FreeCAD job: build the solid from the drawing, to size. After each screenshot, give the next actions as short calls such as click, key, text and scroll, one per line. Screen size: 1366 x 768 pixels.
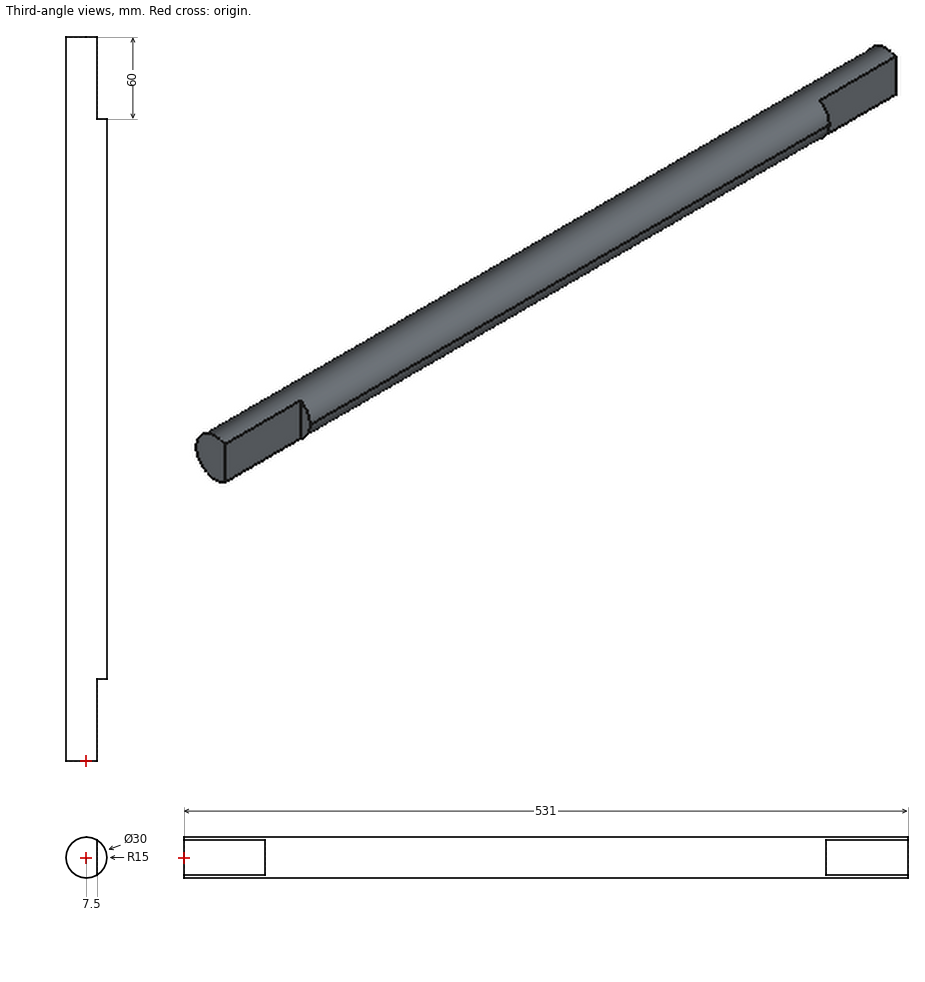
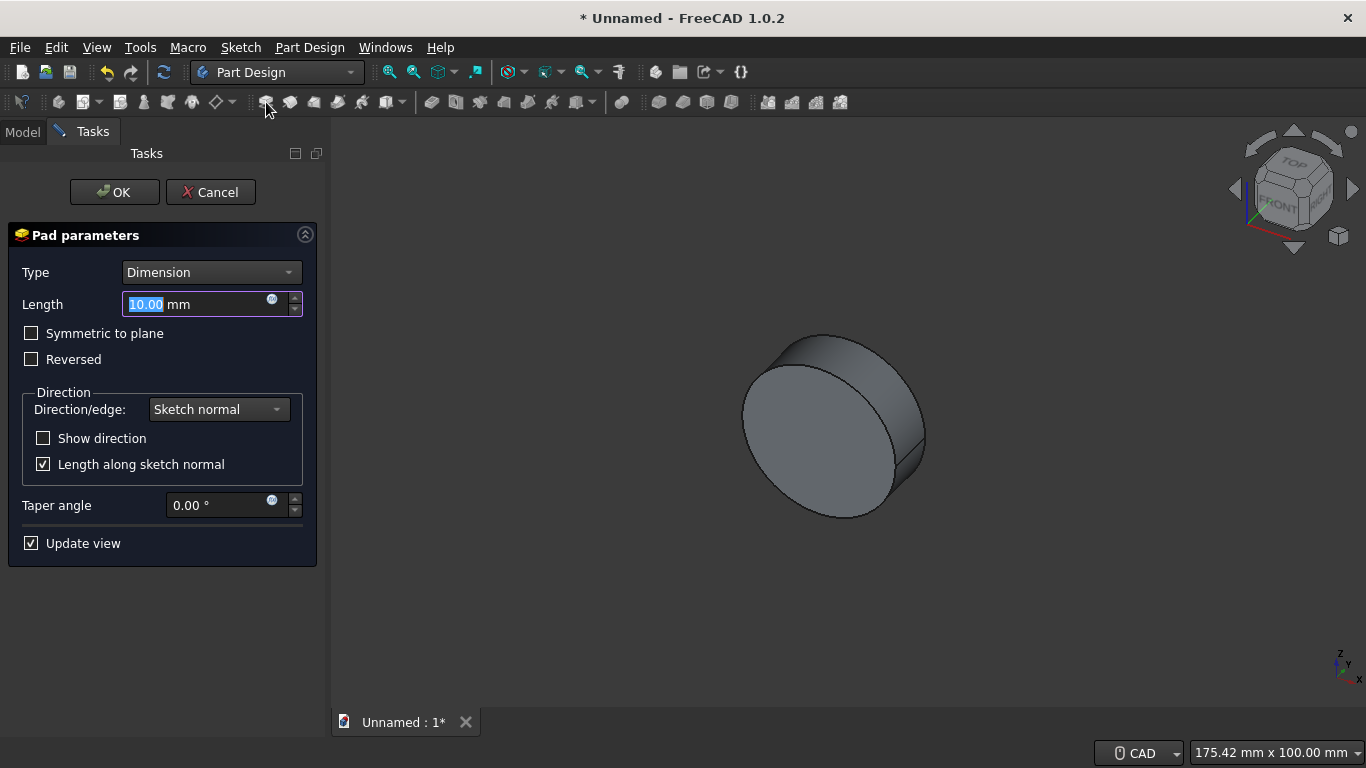
text(531)
key(Tab)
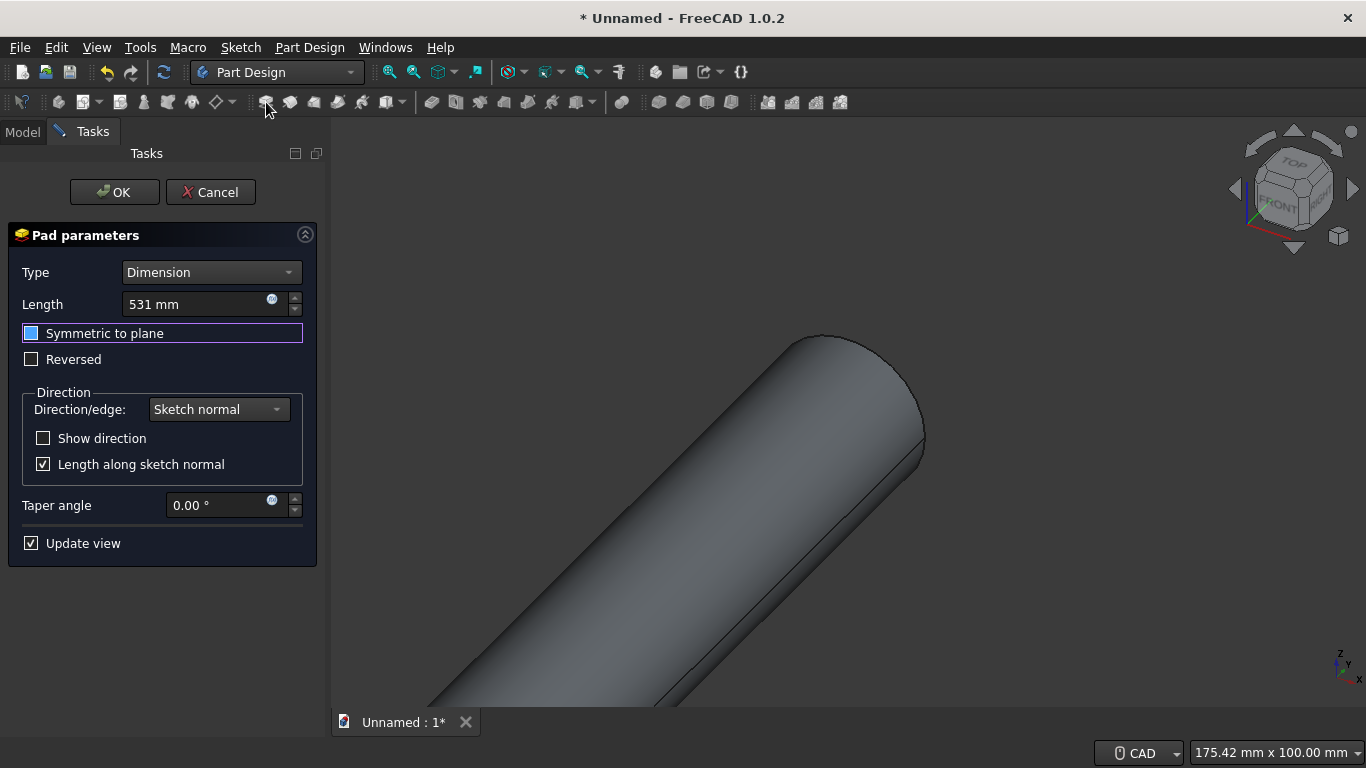
click(30, 359)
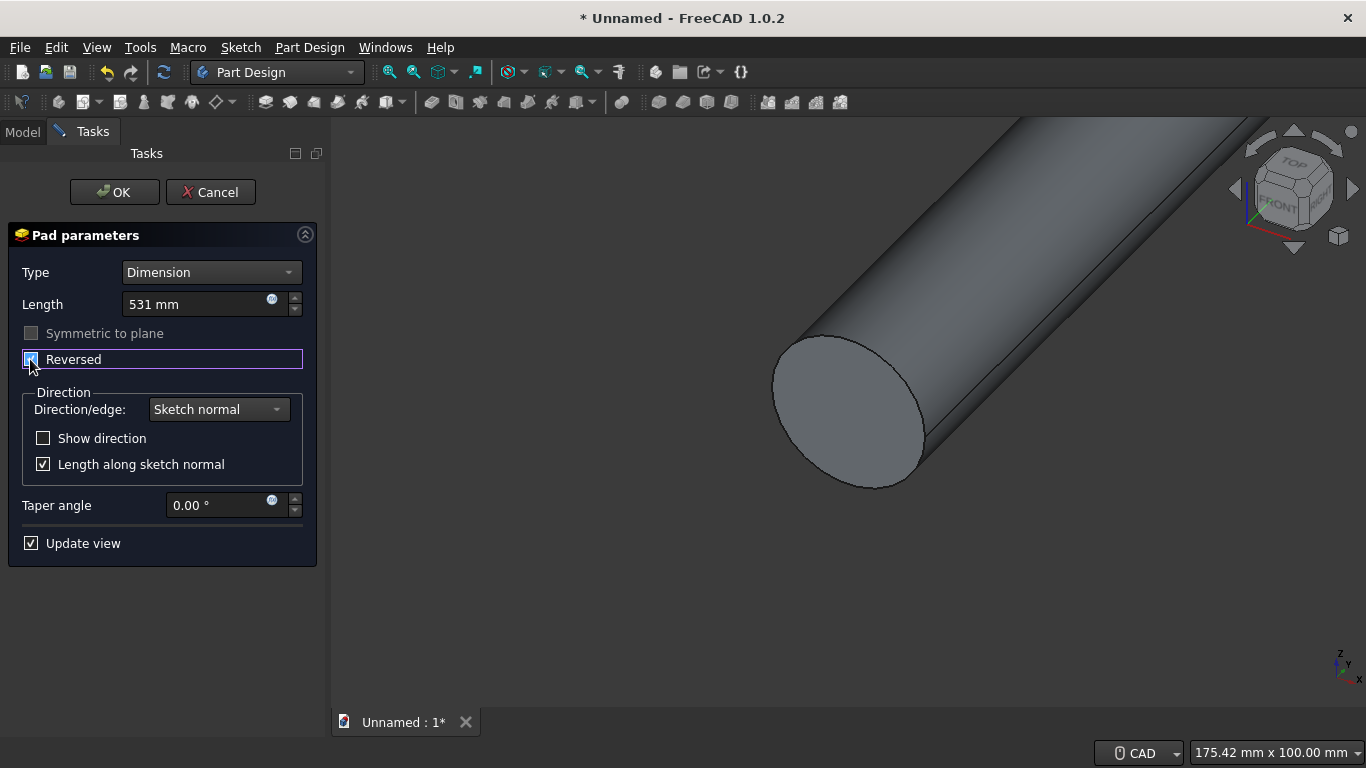
click(115, 192)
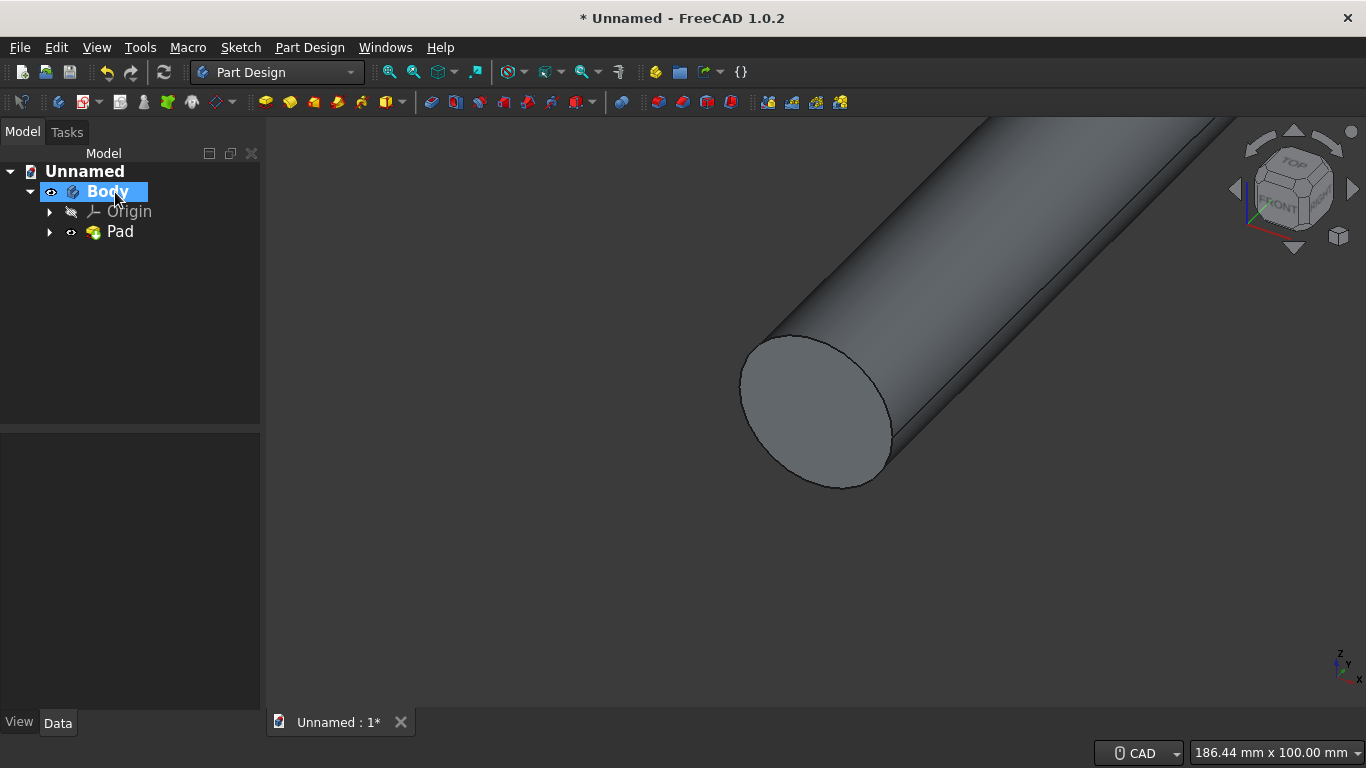
key(v)
key(f)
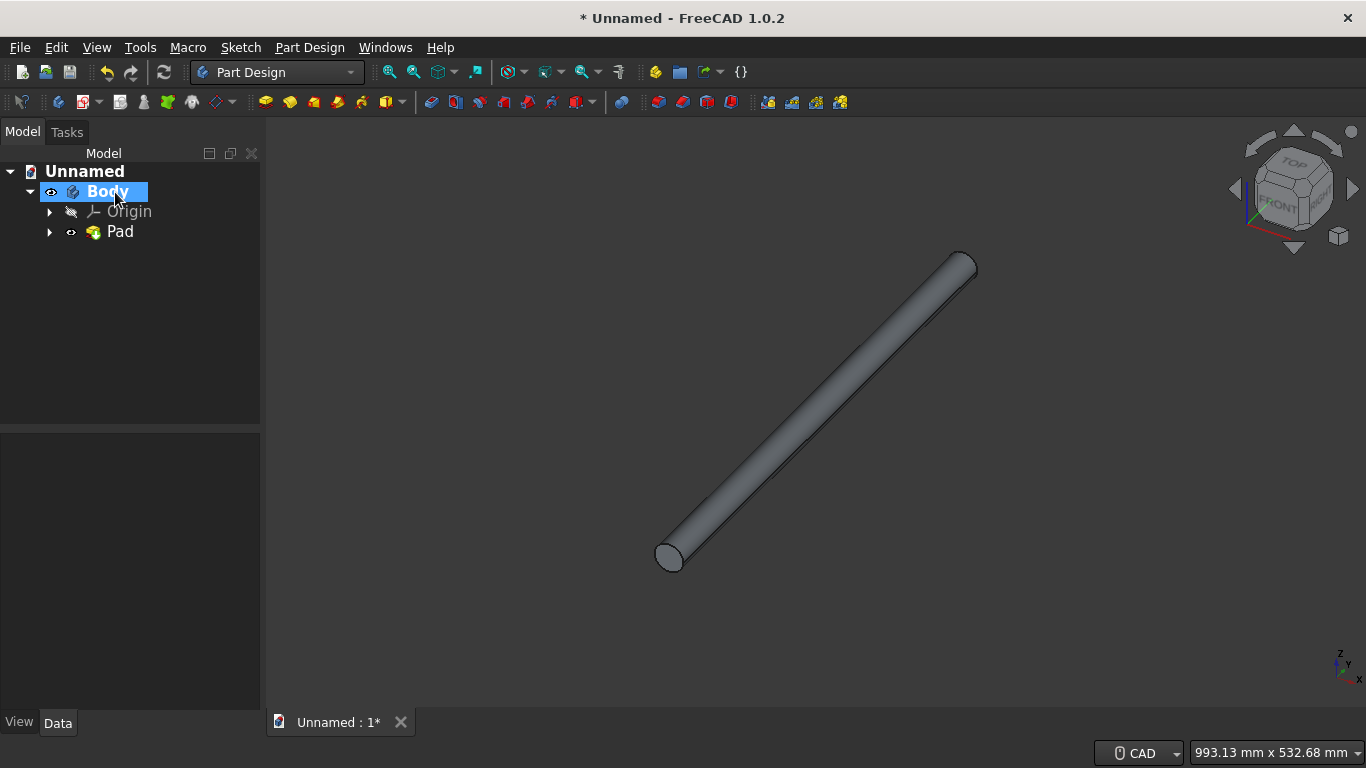
click(50, 212)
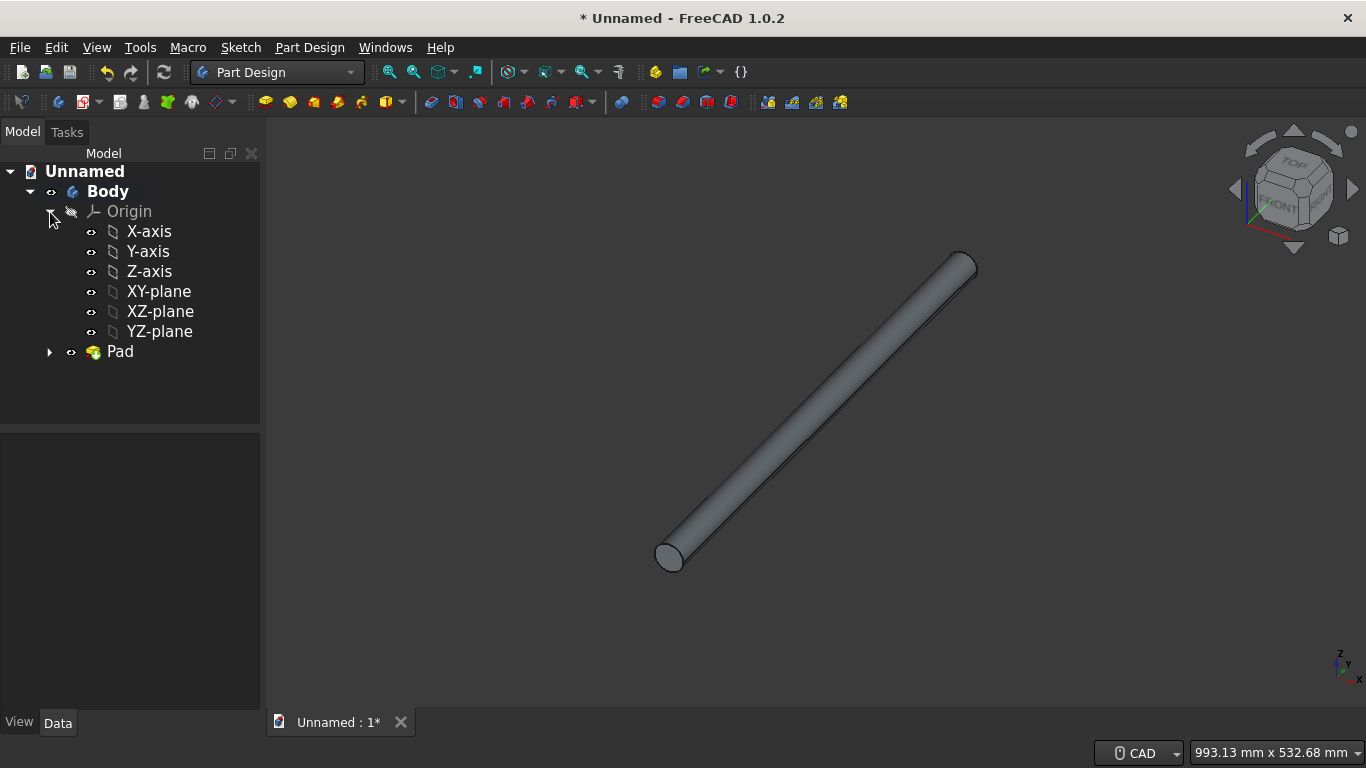
click(136, 312)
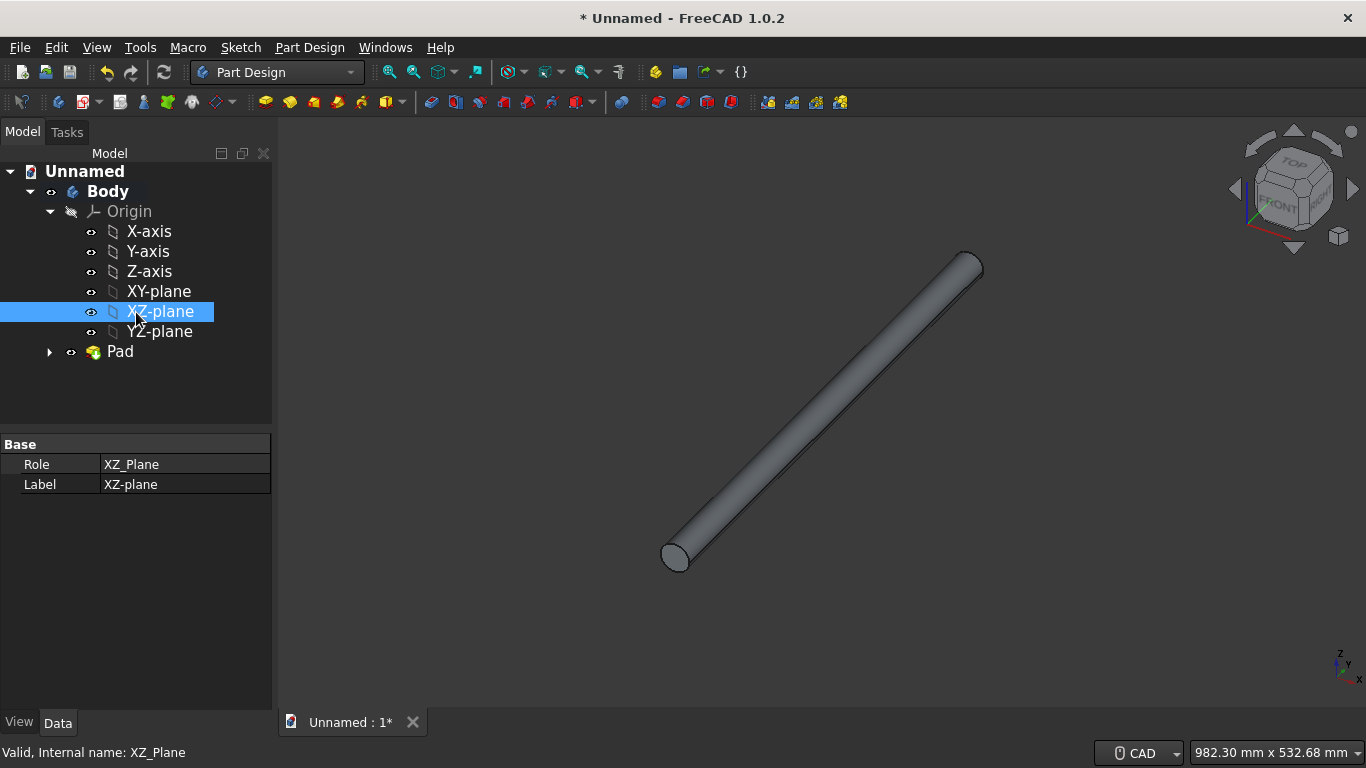
click(216, 102)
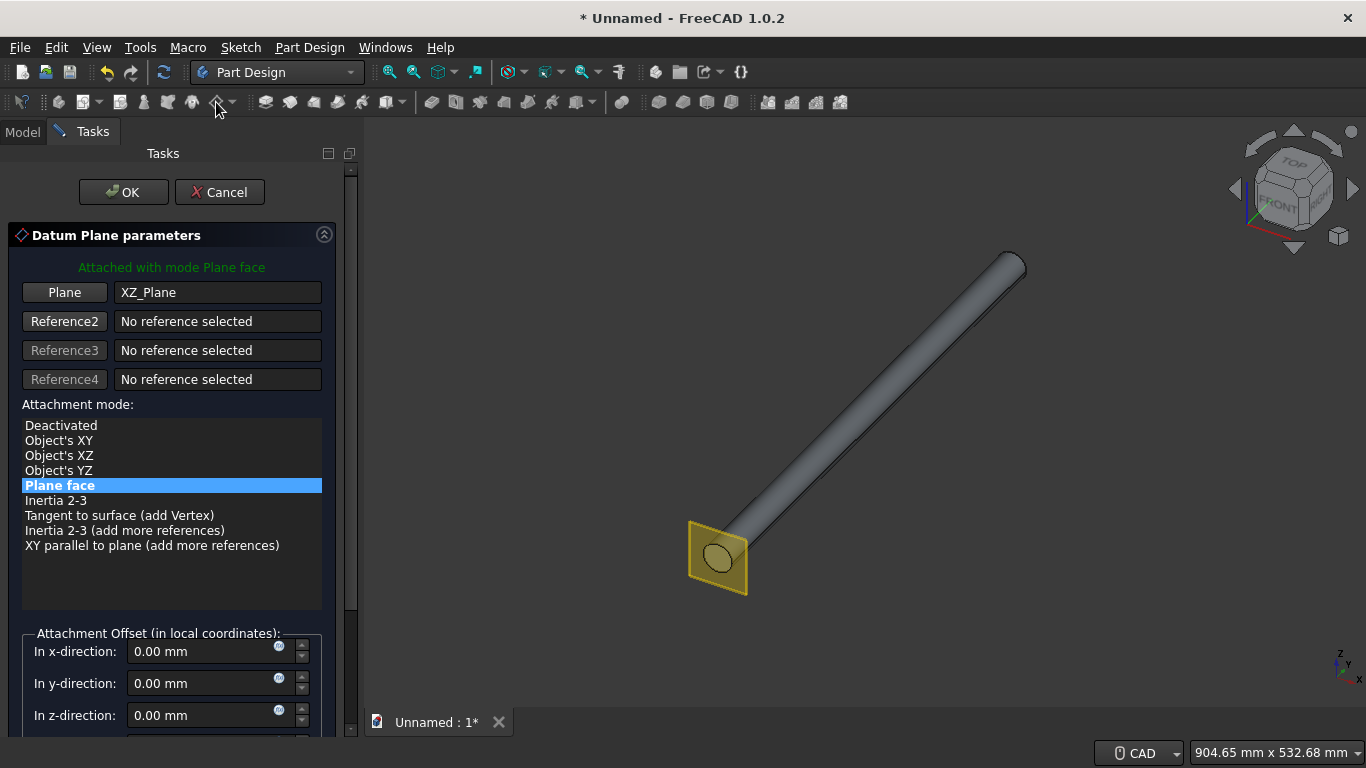
triple_click(210, 715)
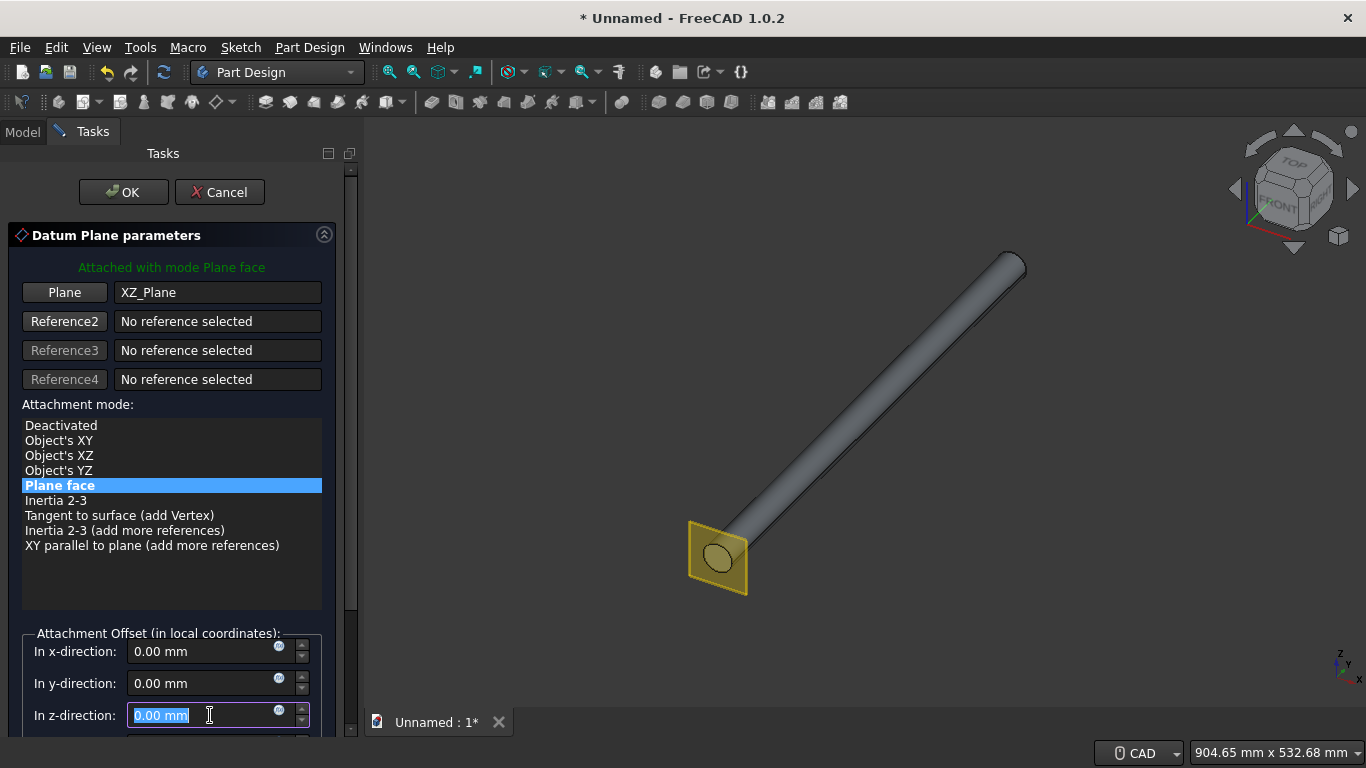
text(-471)
key(Tab)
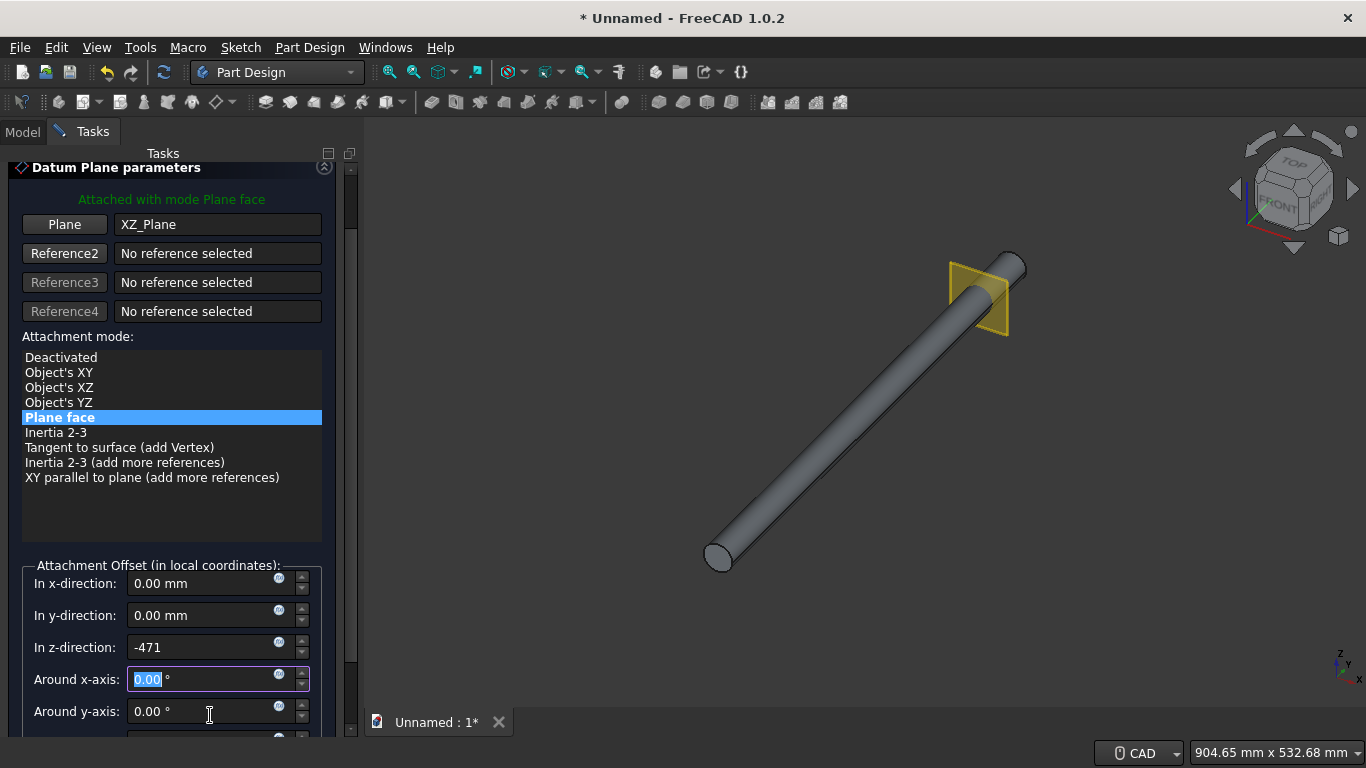
scroll(351, 450, up, 2)